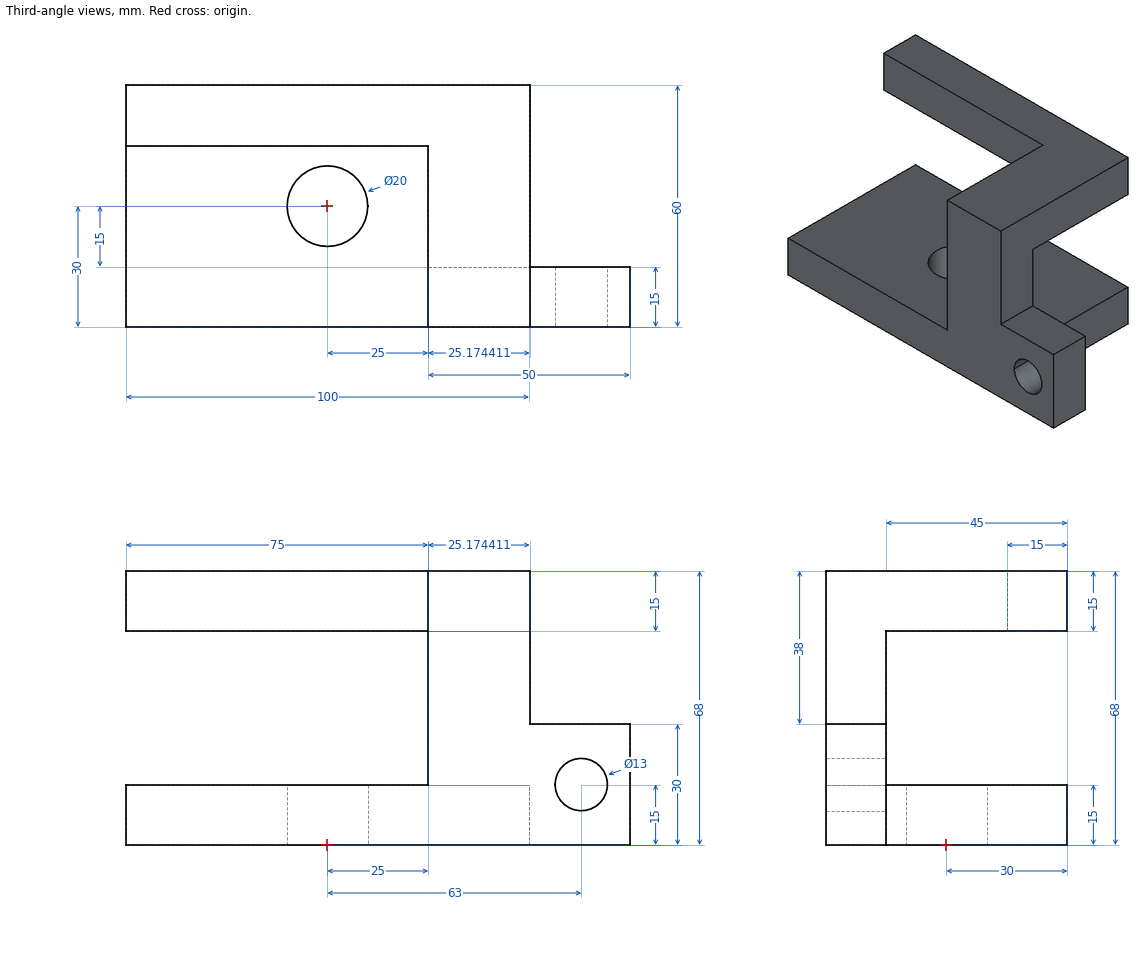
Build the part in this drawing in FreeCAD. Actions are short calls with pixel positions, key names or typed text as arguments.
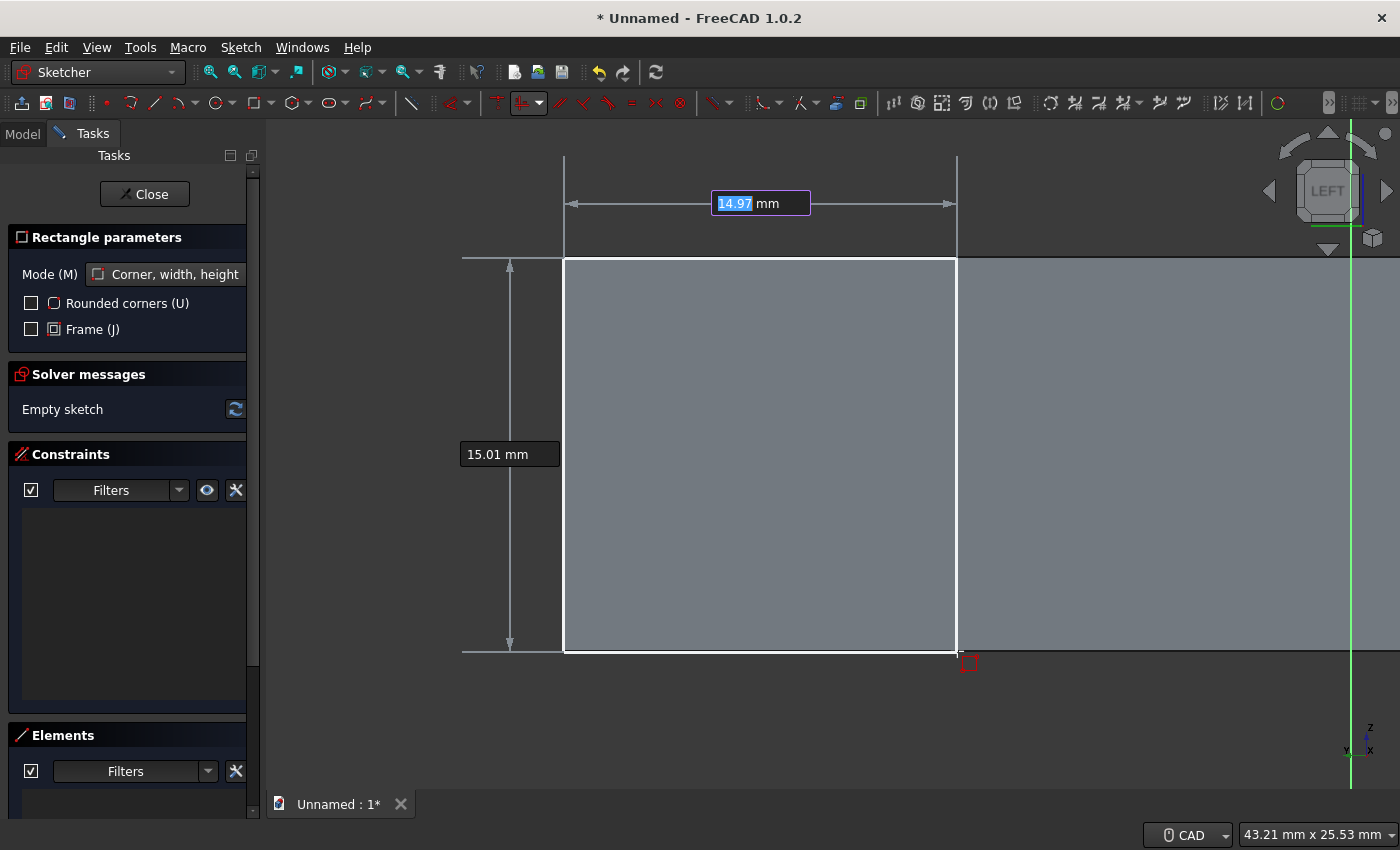
text(15)
key(Tab)
text(15)
key(Return)
key(Escape)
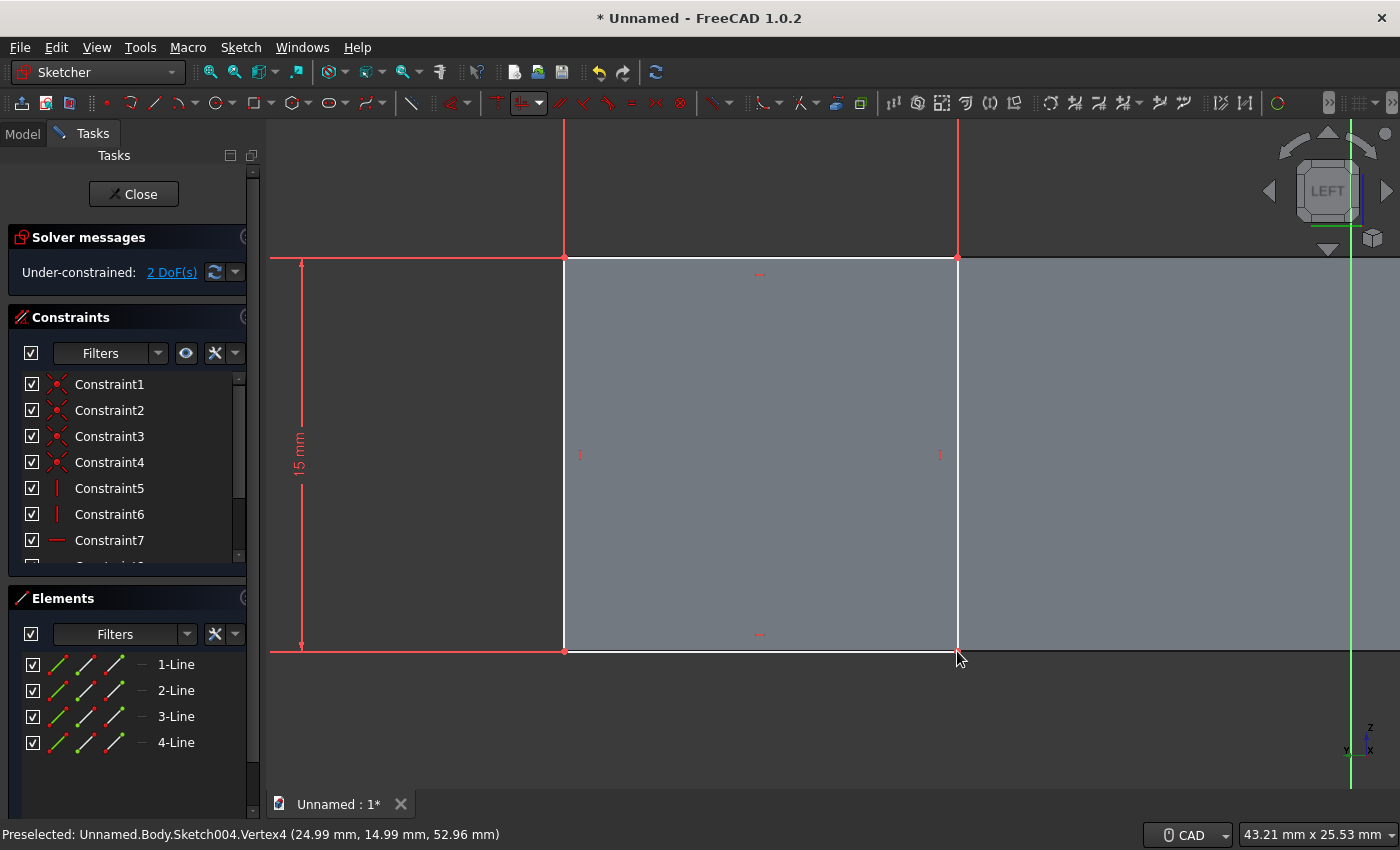
click(450, 104)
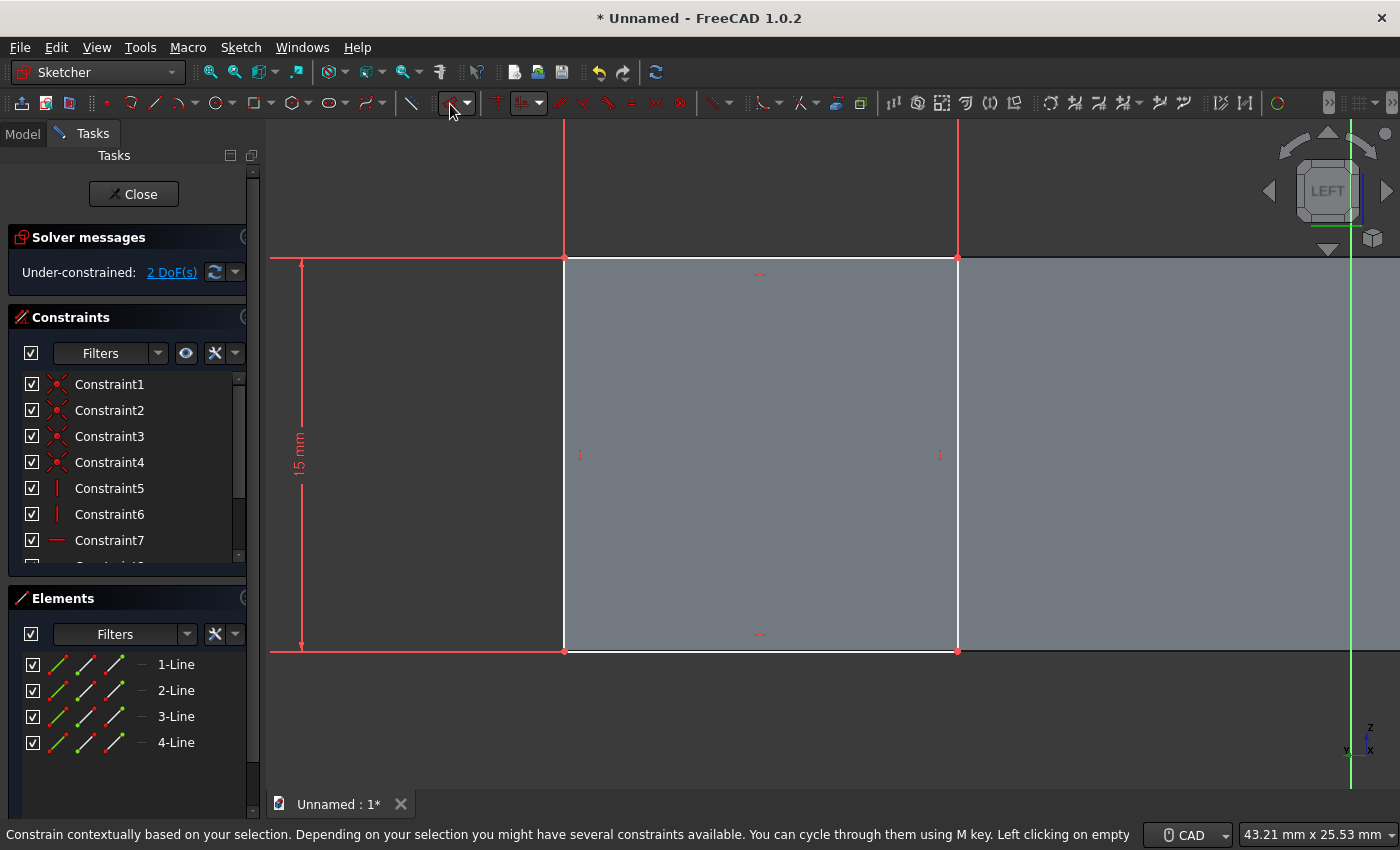
click(564, 258)
click(900, 224)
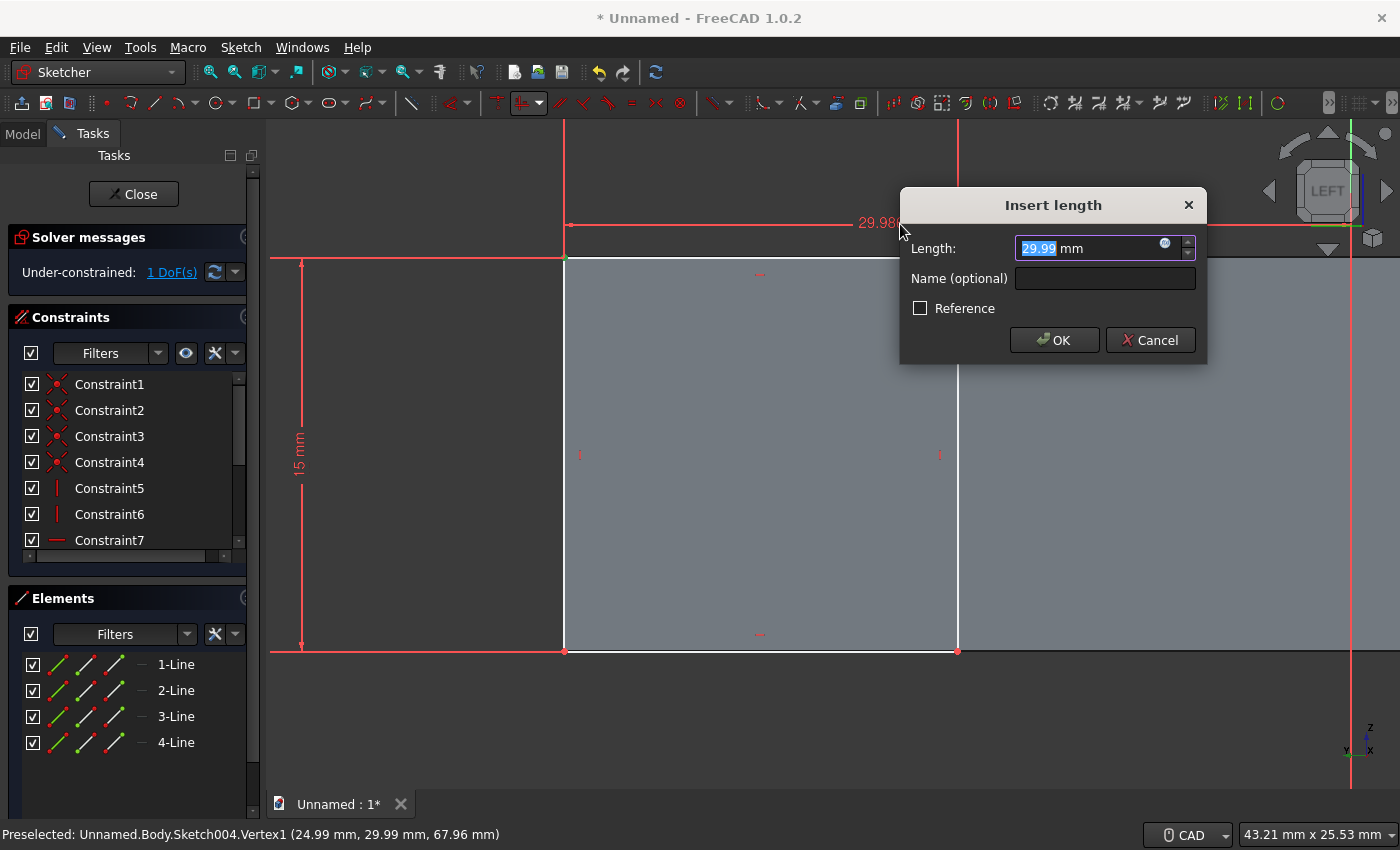
text(30)
key(Return)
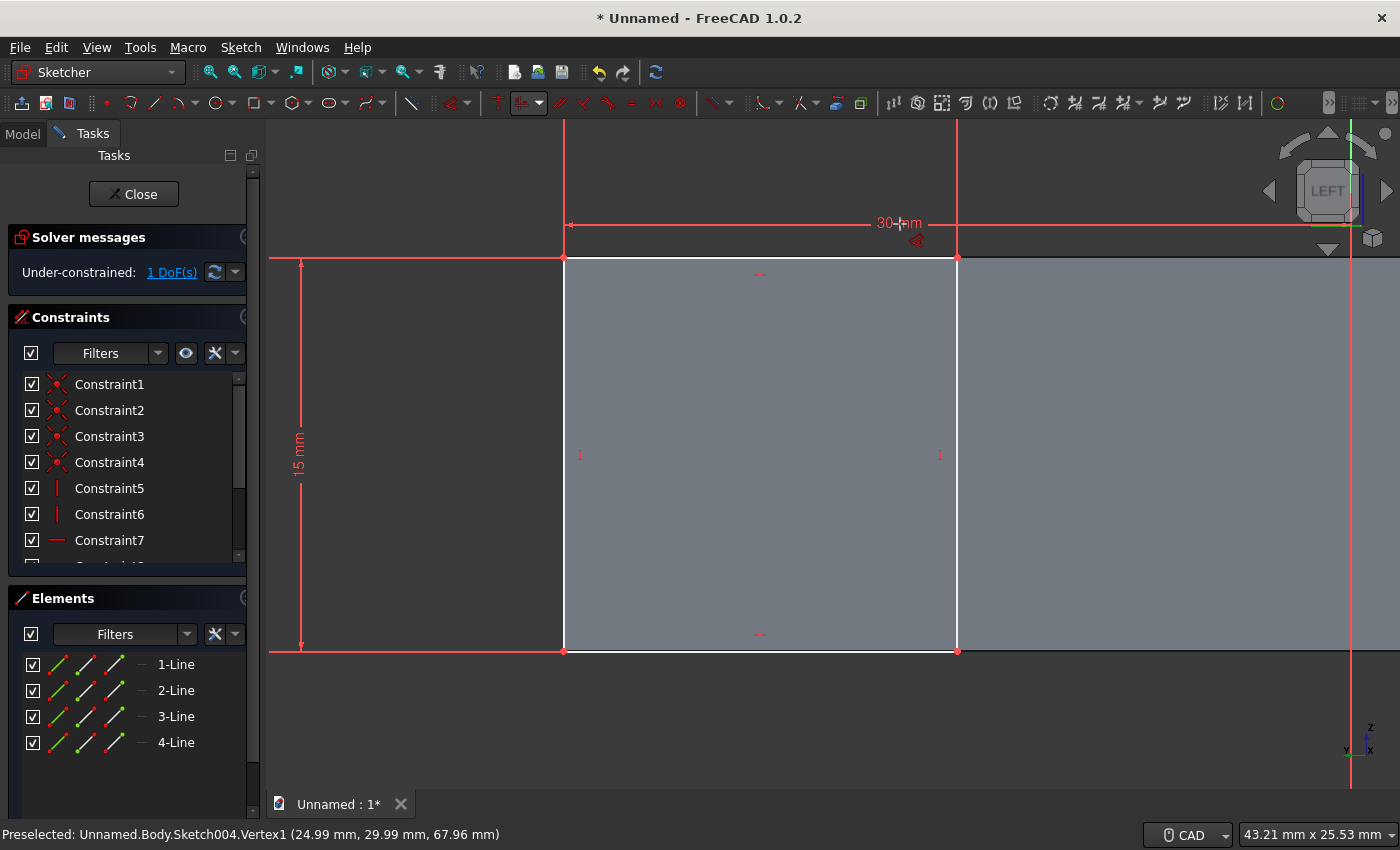
click(564, 258)
click(530, 510)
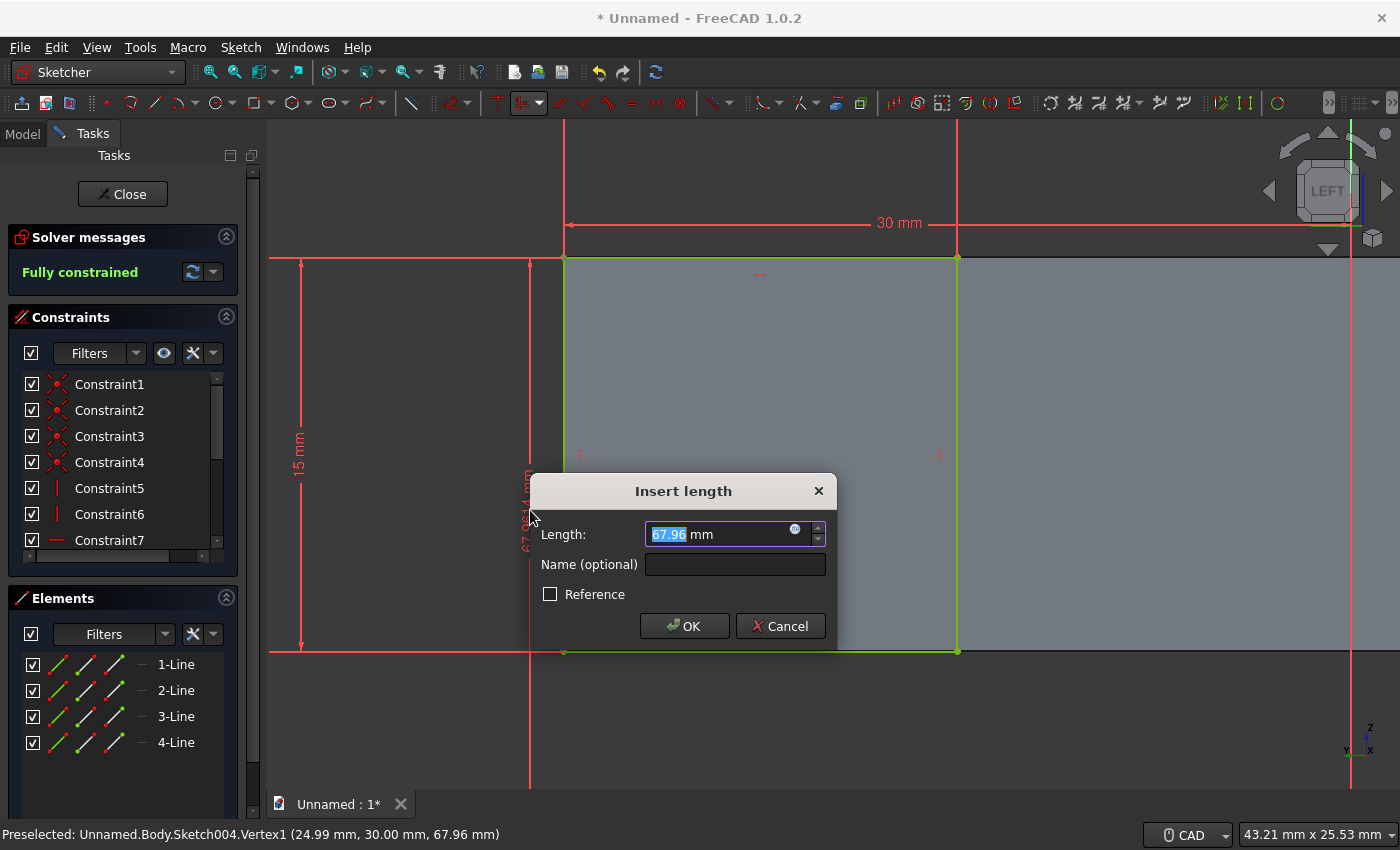
text(68)
key(Return)
key(Escape)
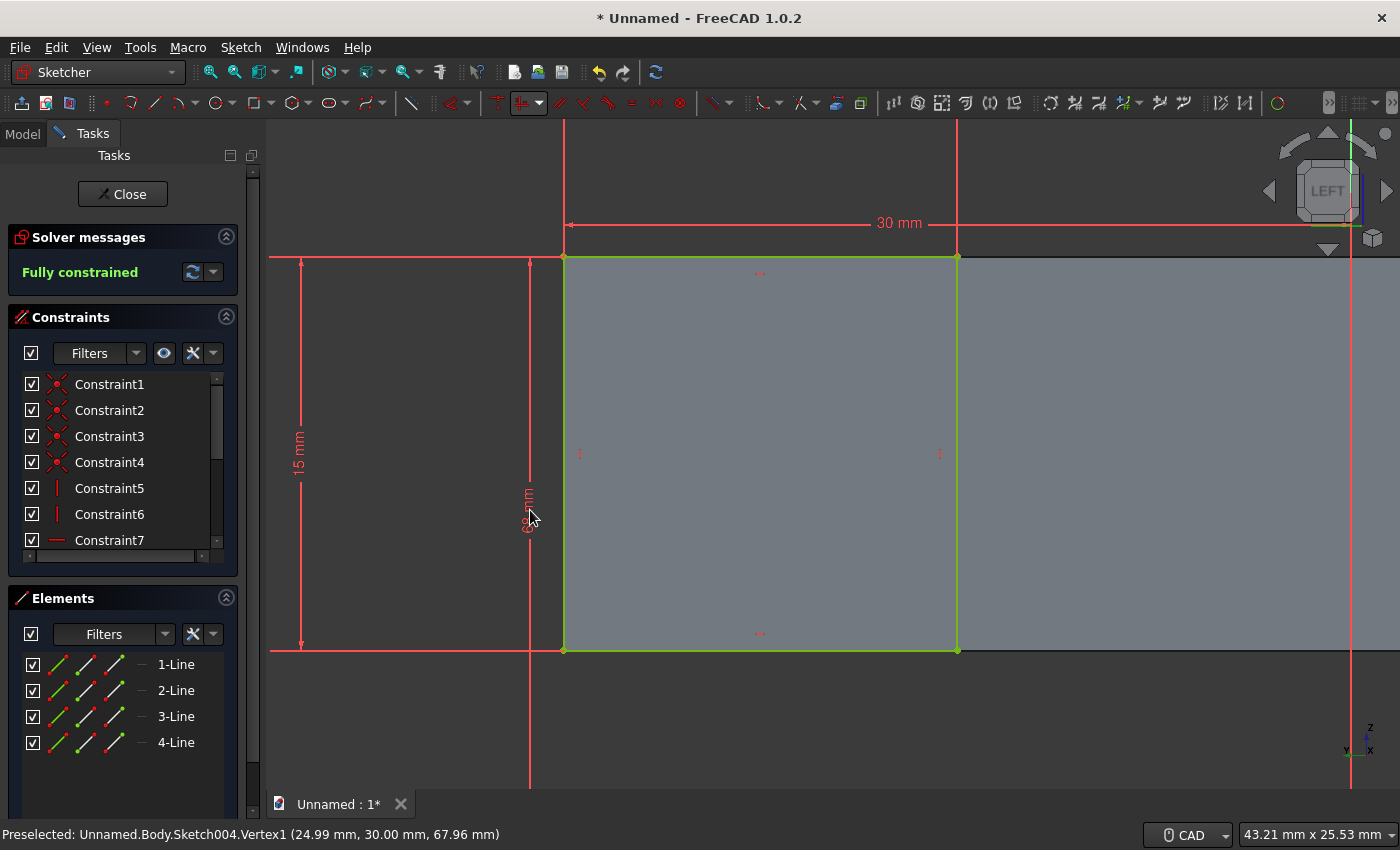
click(123, 194)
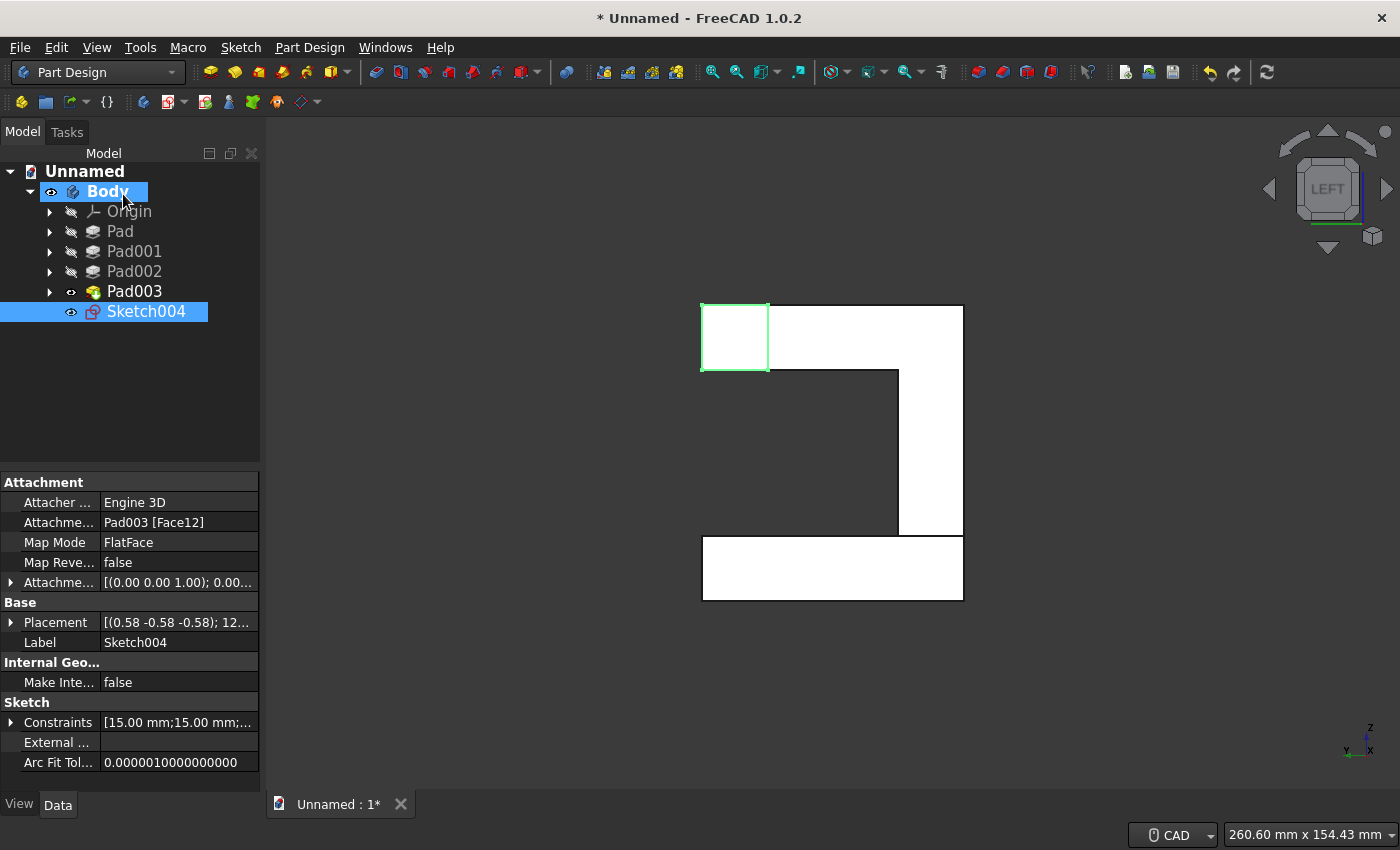
click(212, 72)